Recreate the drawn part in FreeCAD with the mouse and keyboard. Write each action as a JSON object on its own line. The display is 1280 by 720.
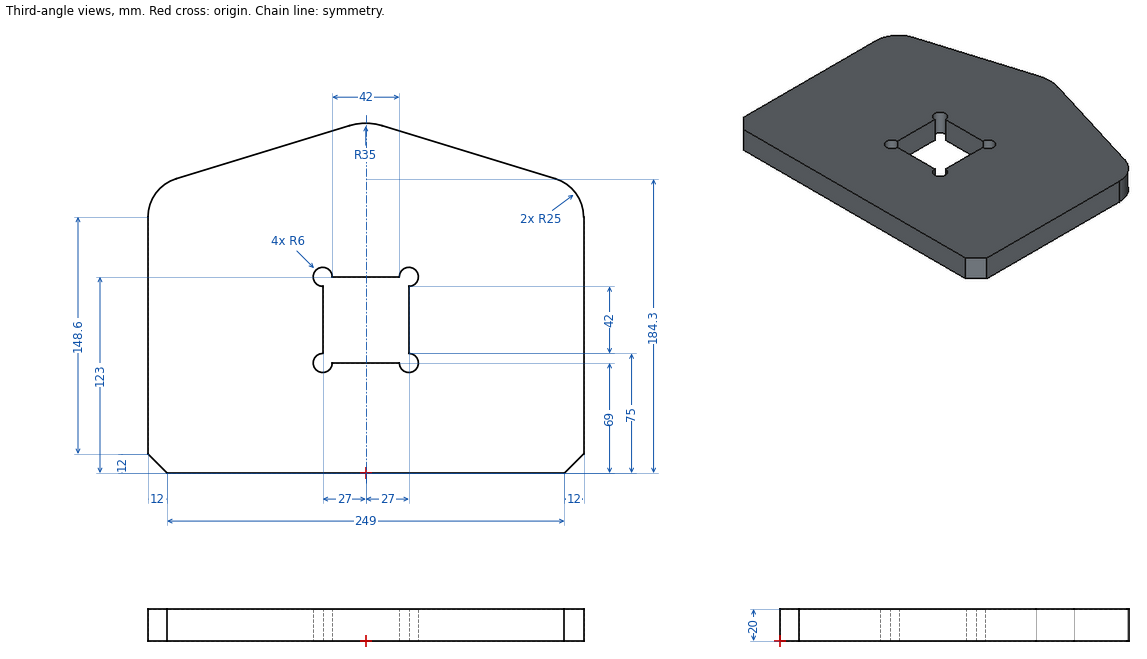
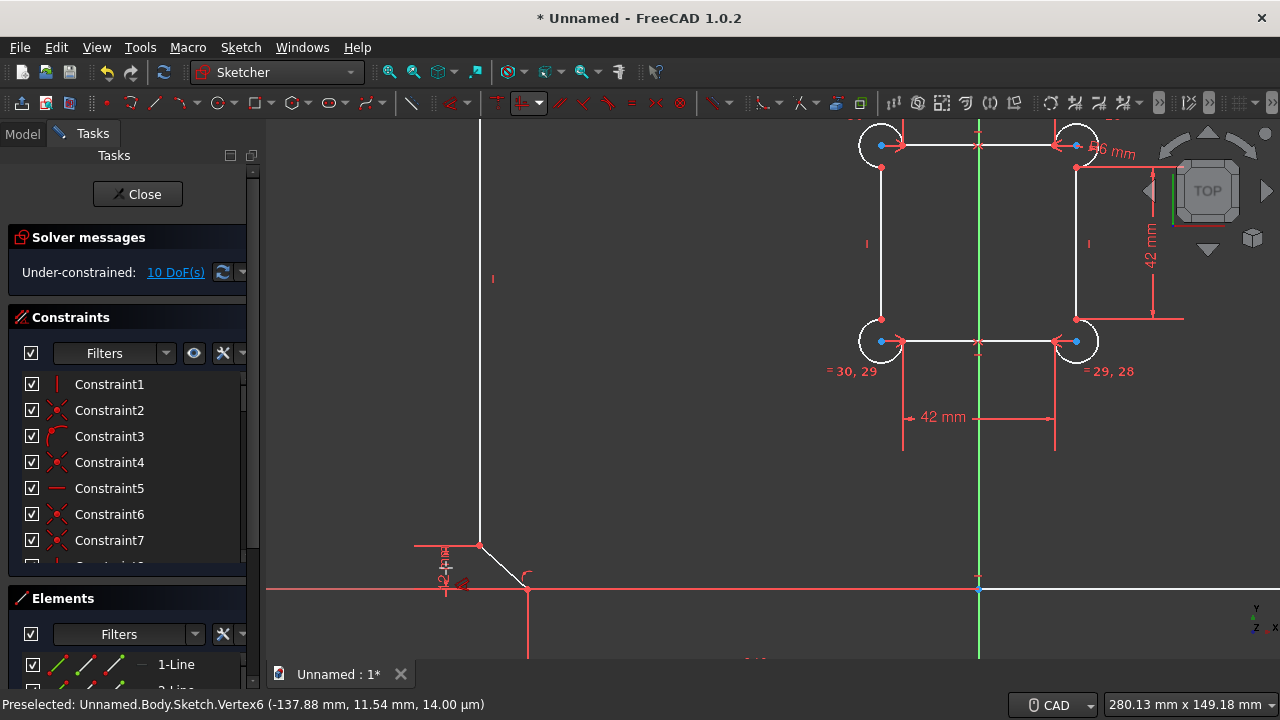
{"action": "scroll", "coordinate": [481, 550], "scroll_direction": "down", "scroll_amount": 4}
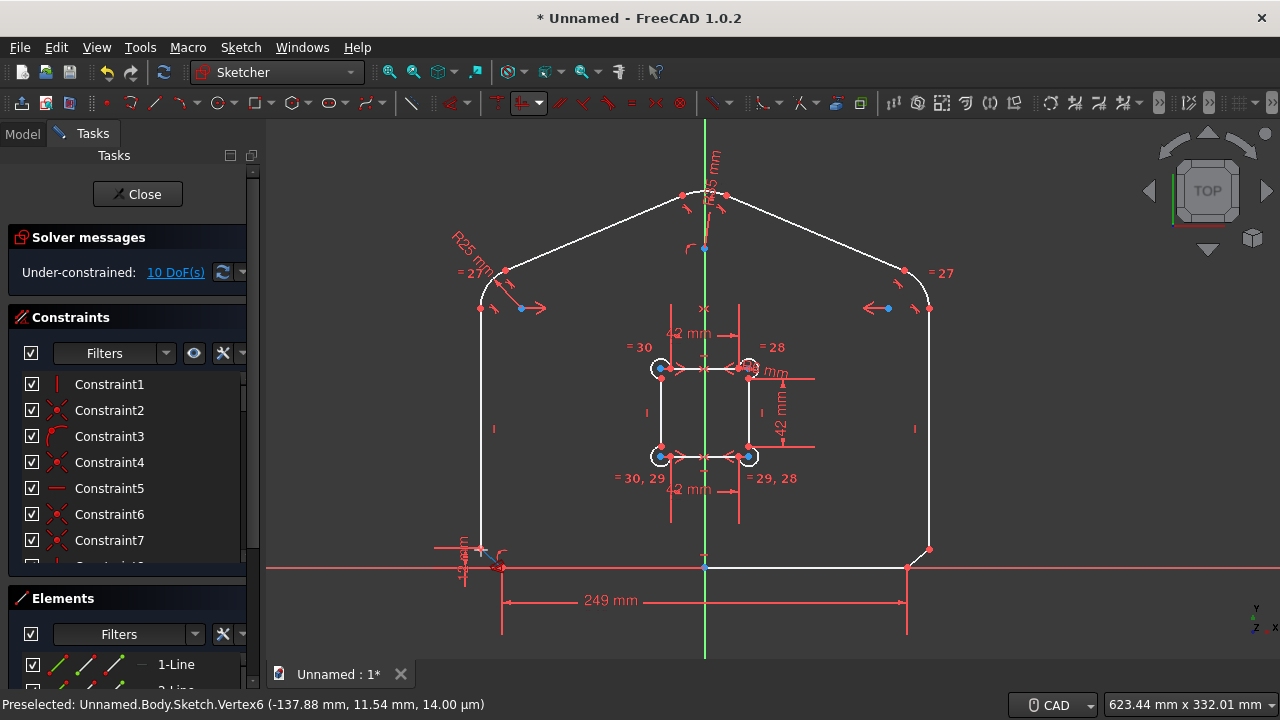
{"action": "scroll", "coordinate": [929, 549], "scroll_direction": "up", "scroll_amount": 4}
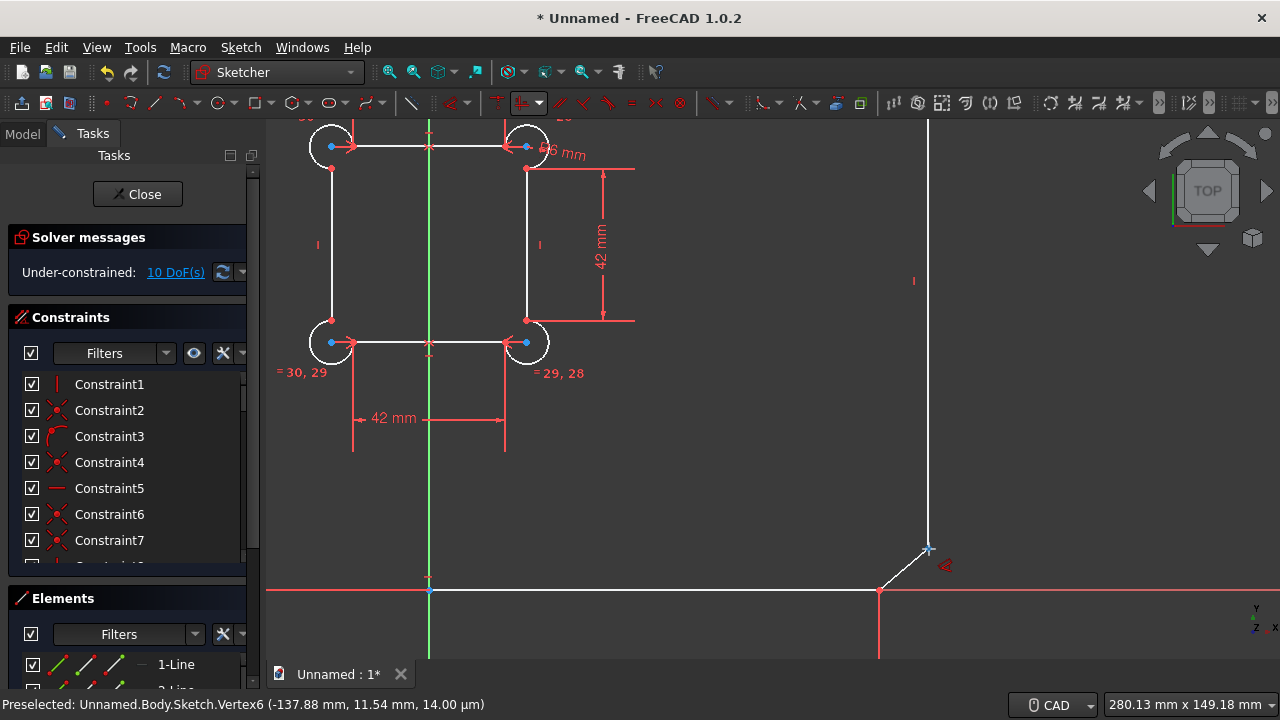
{"action": "left_click", "coordinate": [928, 548]}
{"action": "left_click", "coordinate": [962, 569]}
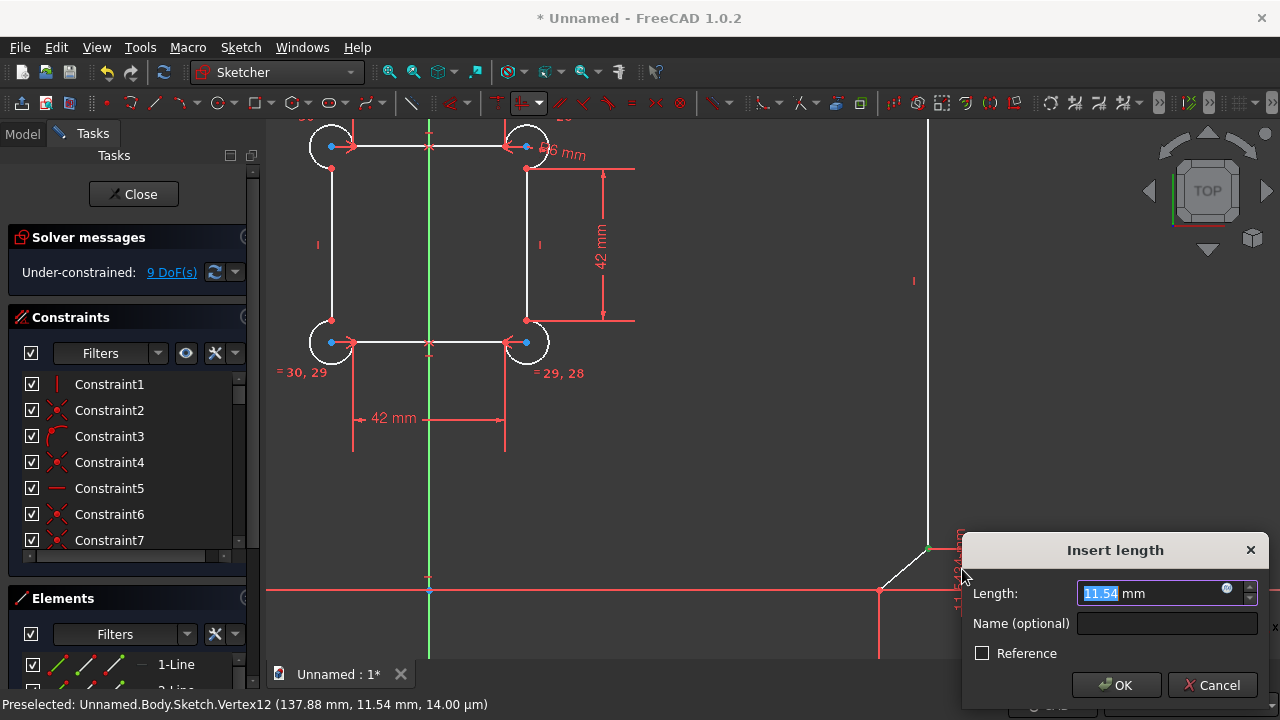
{"action": "type", "text": "12"}
{"action": "key", "text": "Return"}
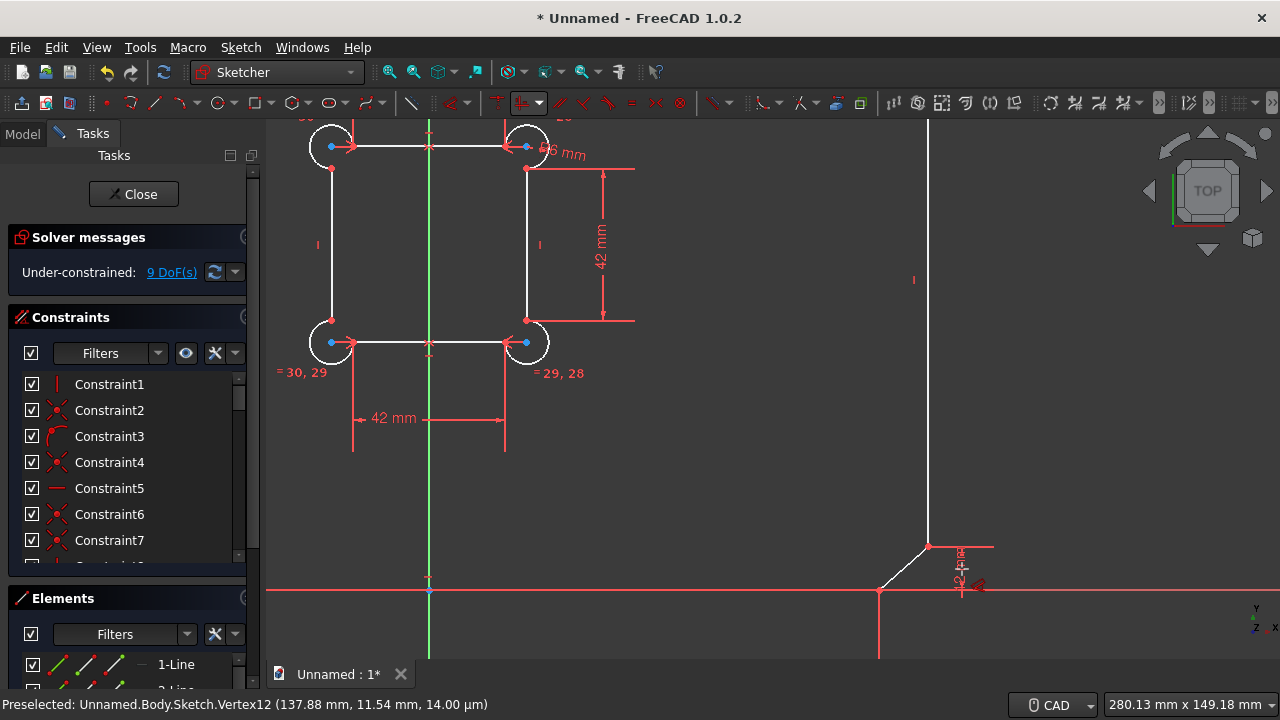
{"action": "left_click", "coordinate": [527, 169]}
{"action": "left_click", "coordinate": [478, 624]}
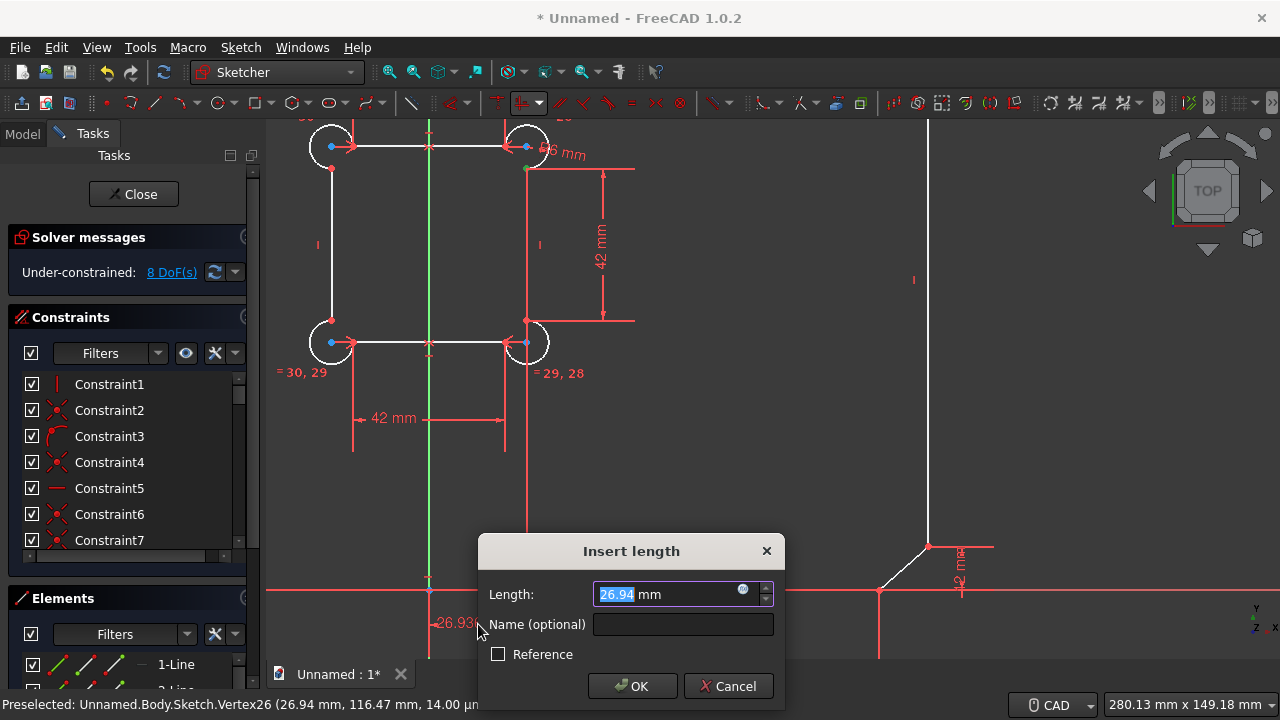
{"action": "type", "text": "27"}
{"action": "key", "text": "Return"}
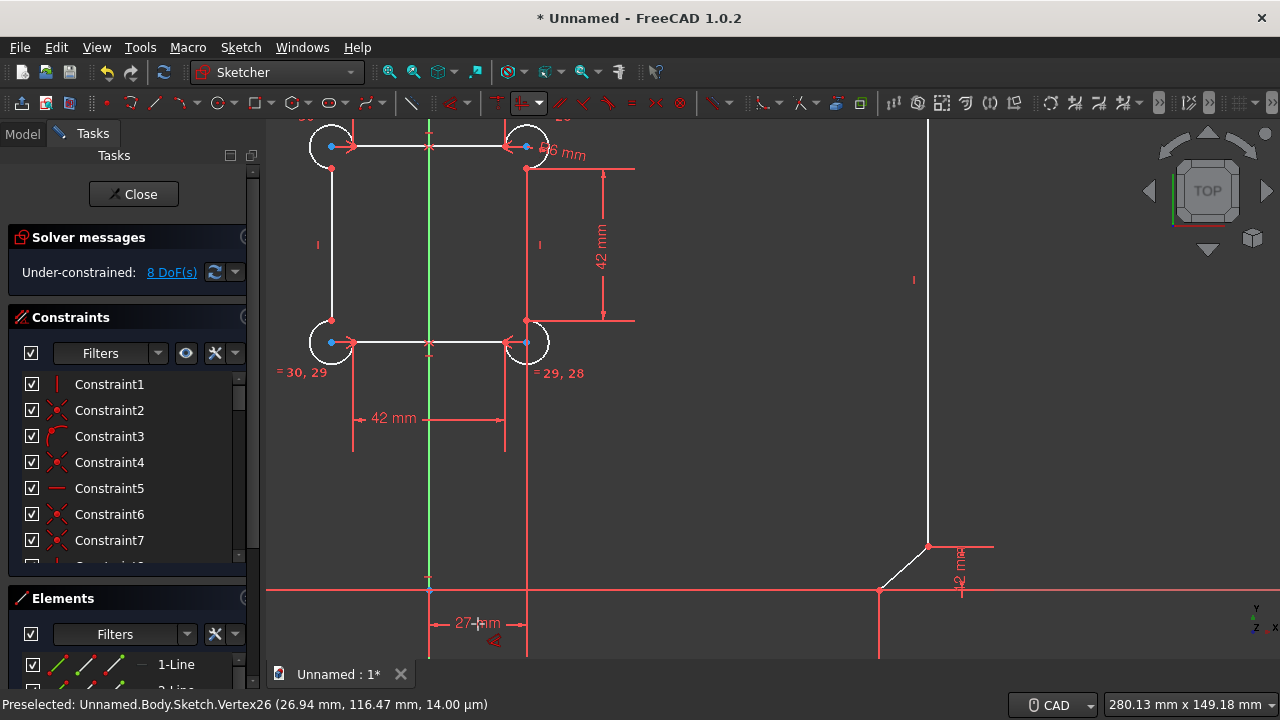
{"action": "left_click", "coordinate": [527, 321]}
{"action": "left_click", "coordinate": [561, 455]}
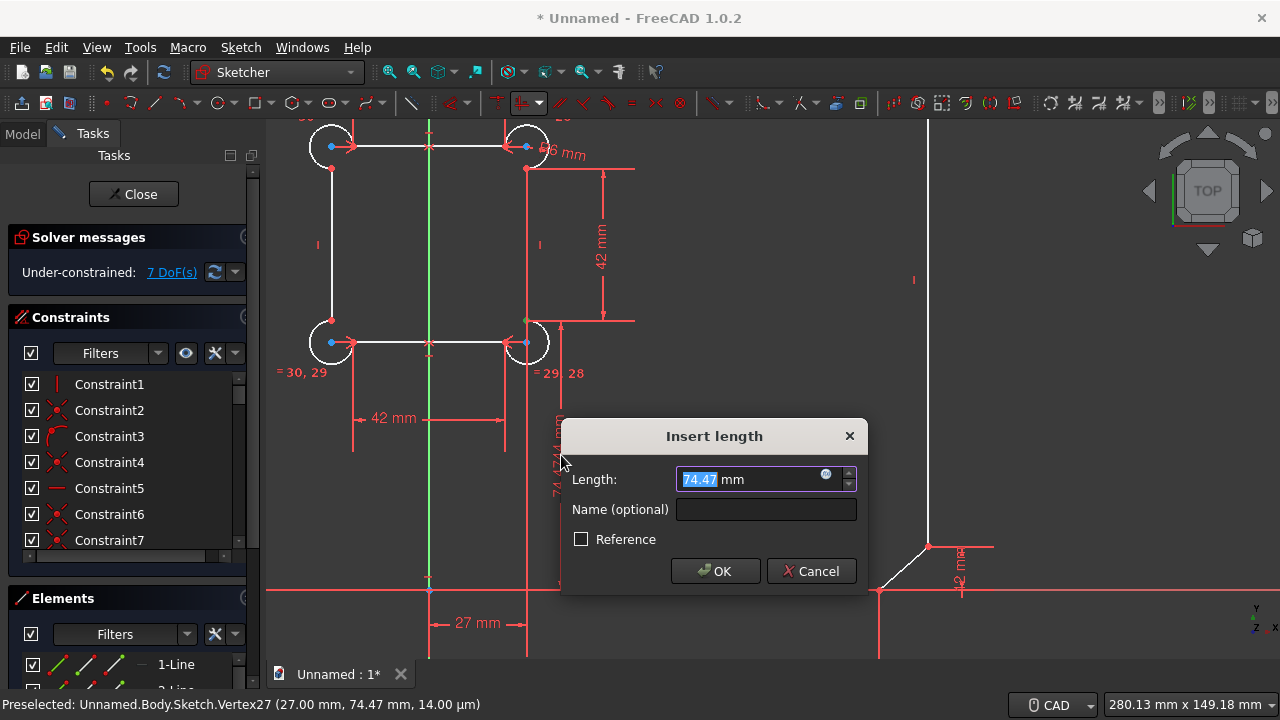
{"action": "type", "text": "75"}
{"action": "key", "text": "Return"}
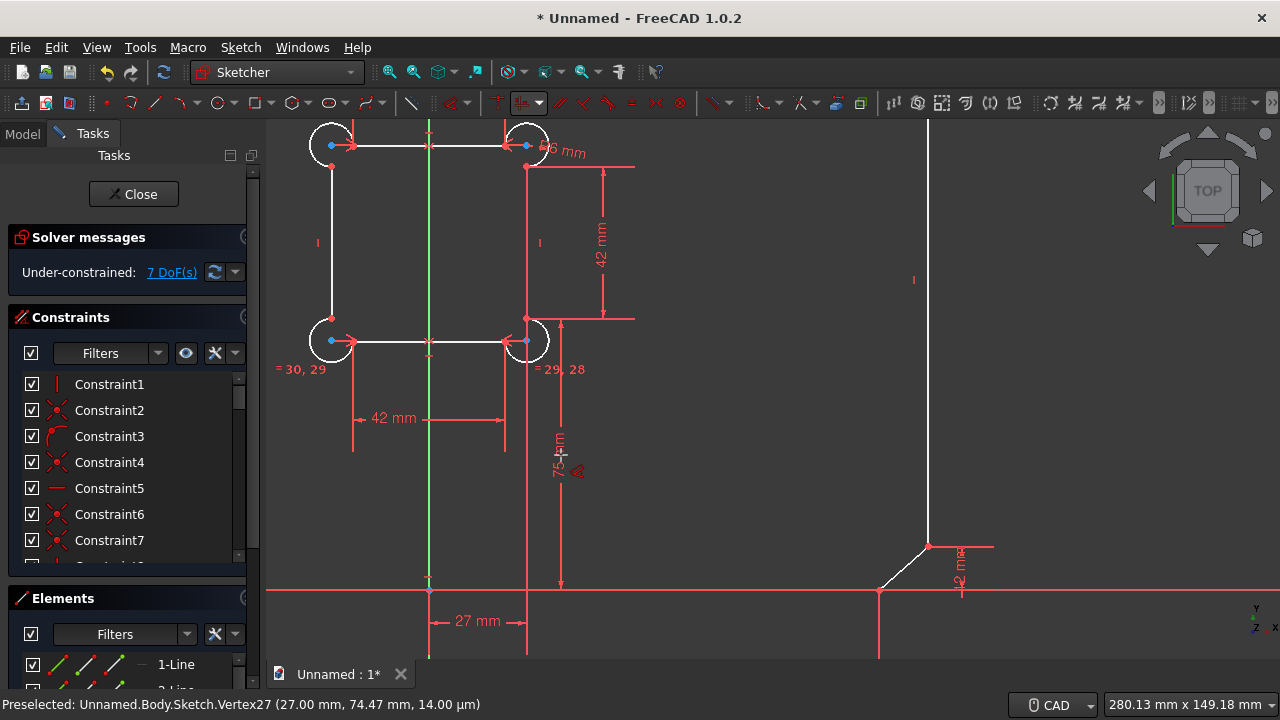
{"action": "left_click", "coordinate": [505, 342]}
{"action": "left_click", "coordinate": [539, 409]}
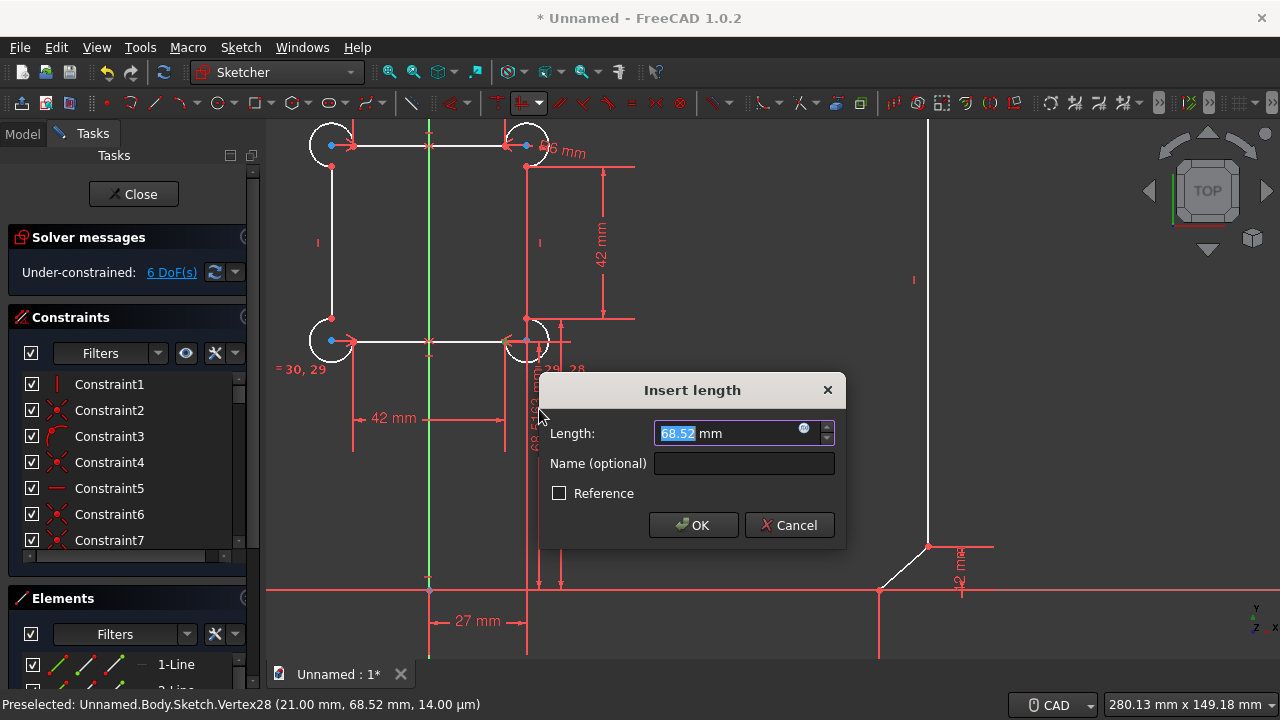
{"action": "type", "text": "69"}
{"action": "key", "text": "Return"}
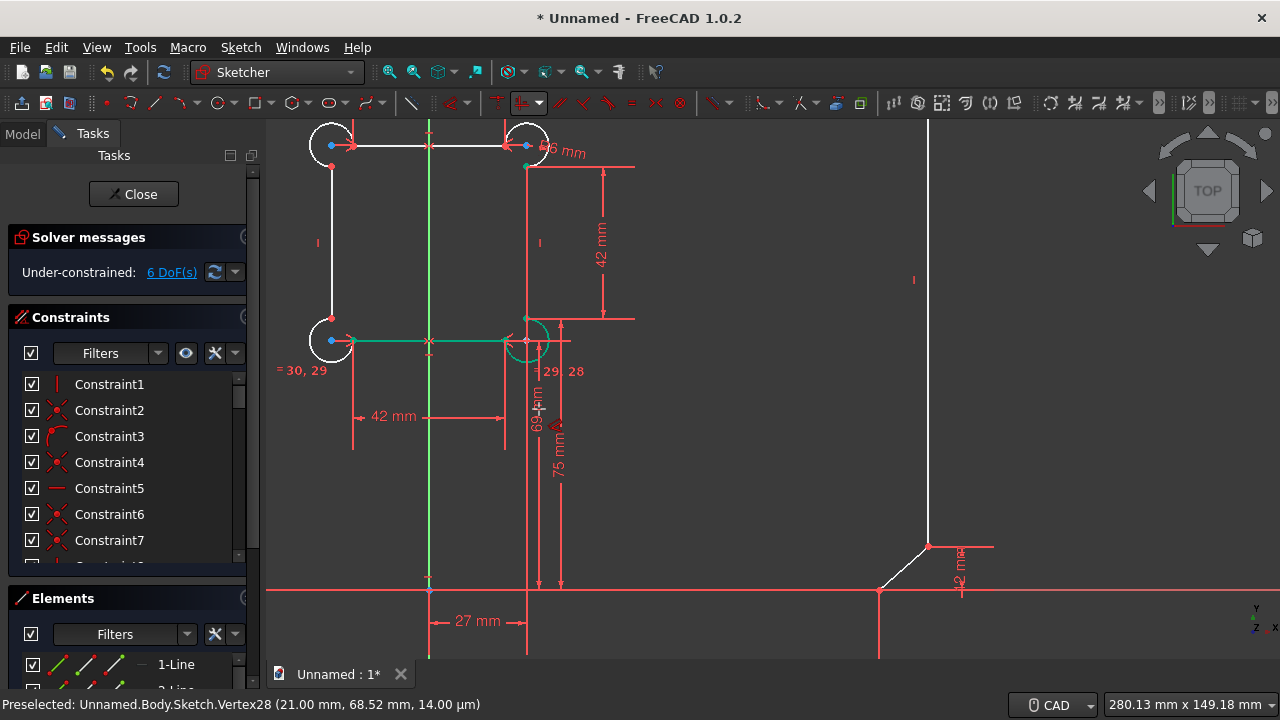
{"action": "left_click", "coordinate": [332, 319]}
{"action": "left_click", "coordinate": [380, 624]}